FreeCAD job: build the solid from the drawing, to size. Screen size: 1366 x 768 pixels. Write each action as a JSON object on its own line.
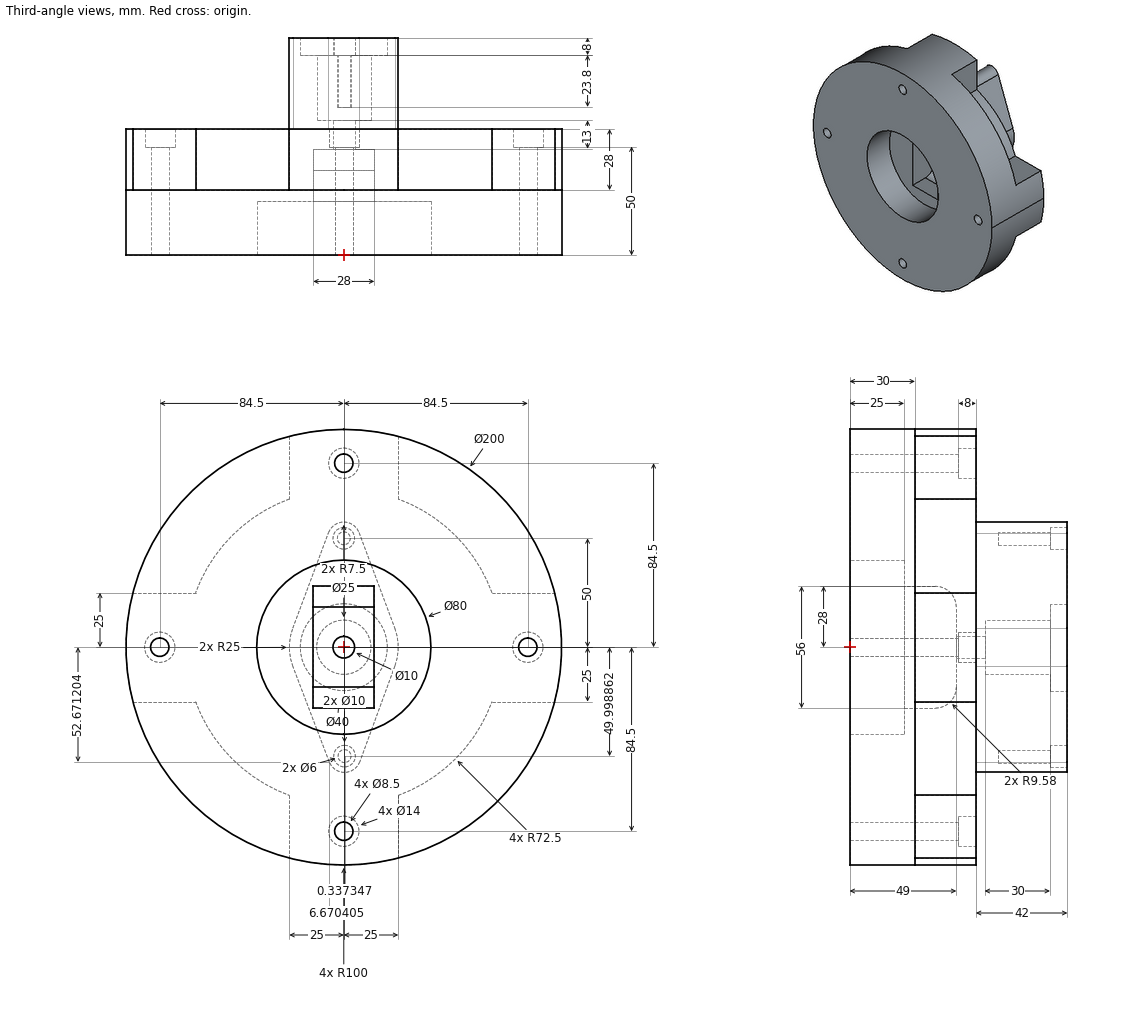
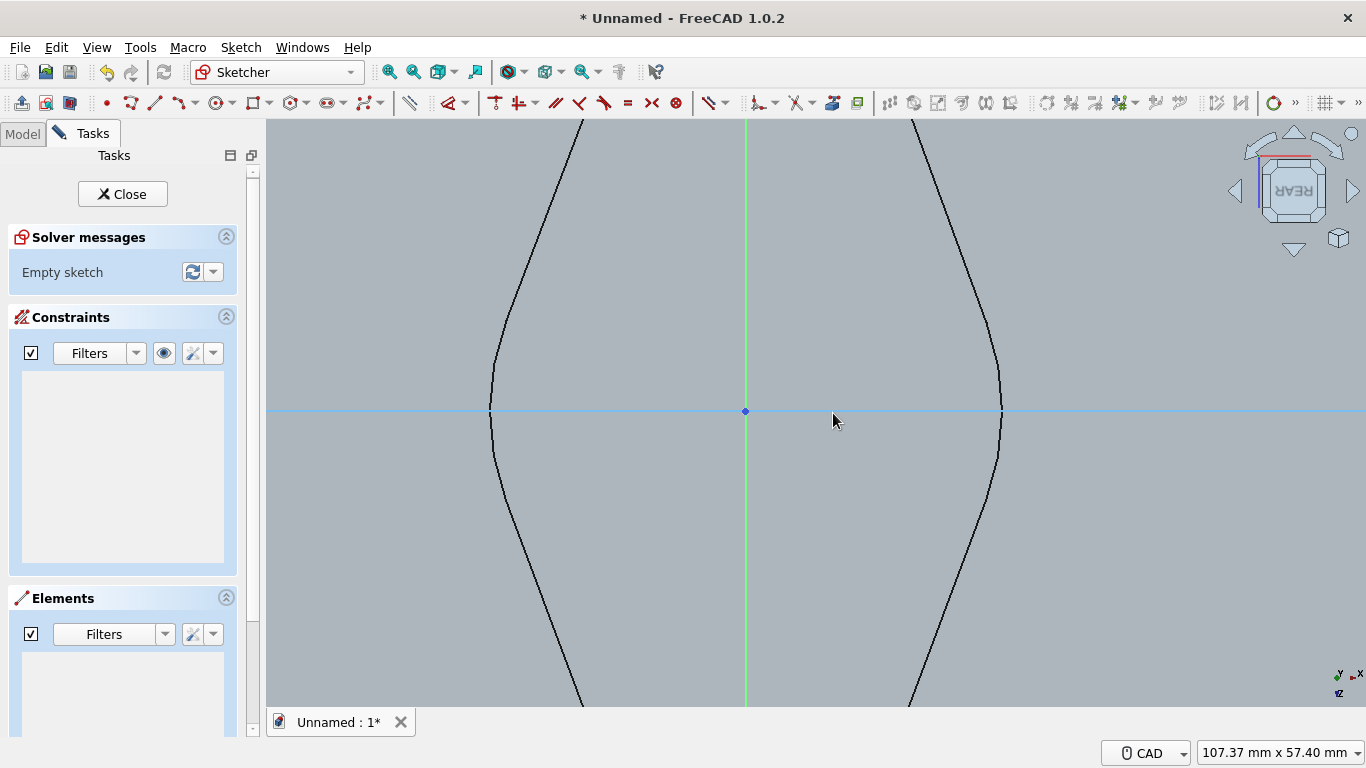
{"action": "key", "text": "g c"}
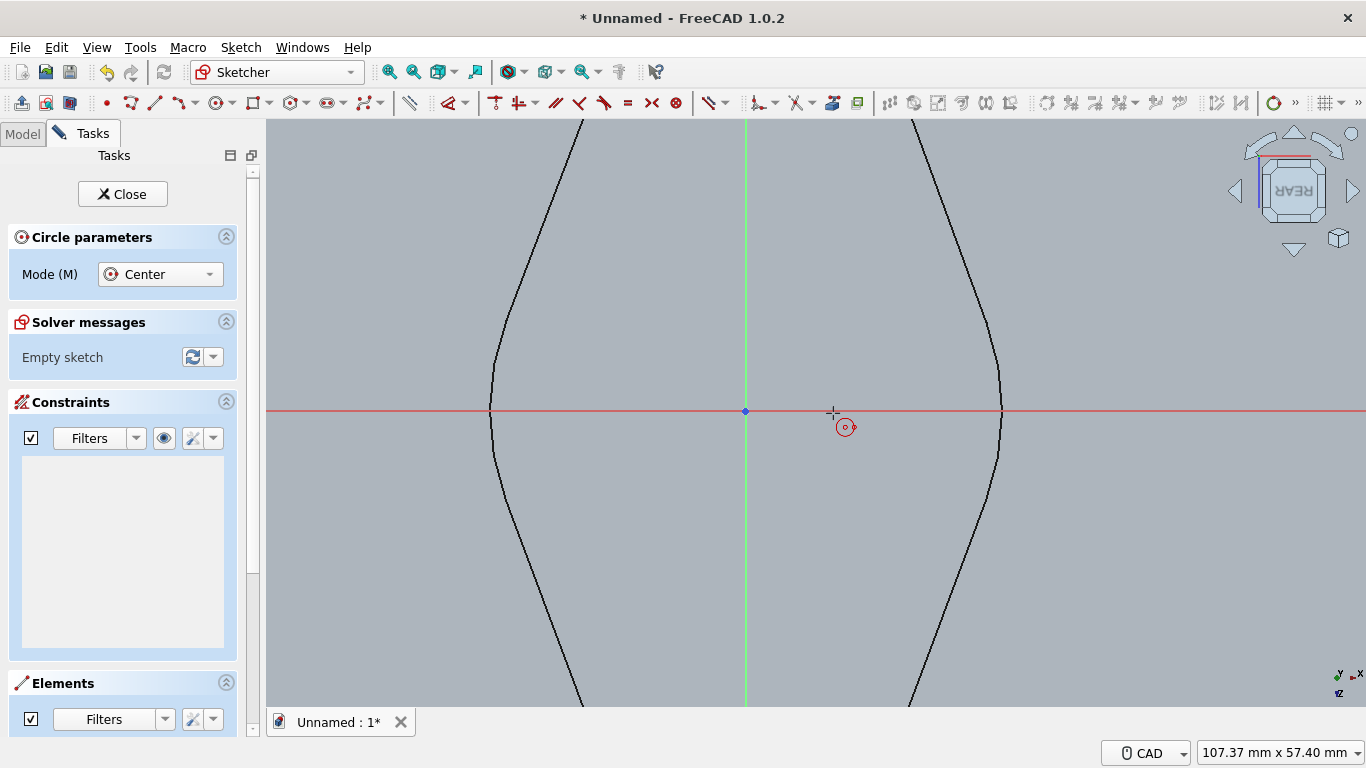
{"action": "left_click", "coordinate": [746, 411]}
{"action": "left_click", "coordinate": [891, 266]}
{"action": "key", "text": "Escape"}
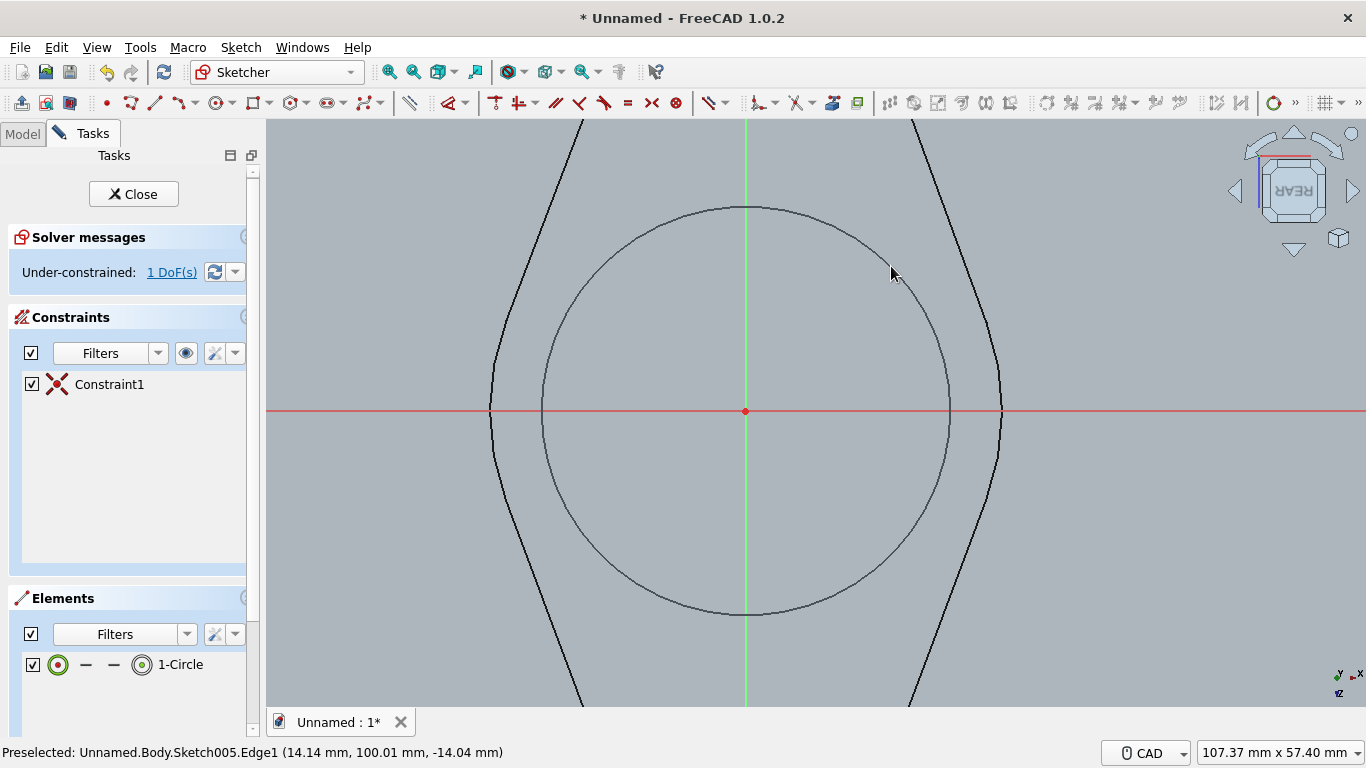
{"action": "key", "text": "d"}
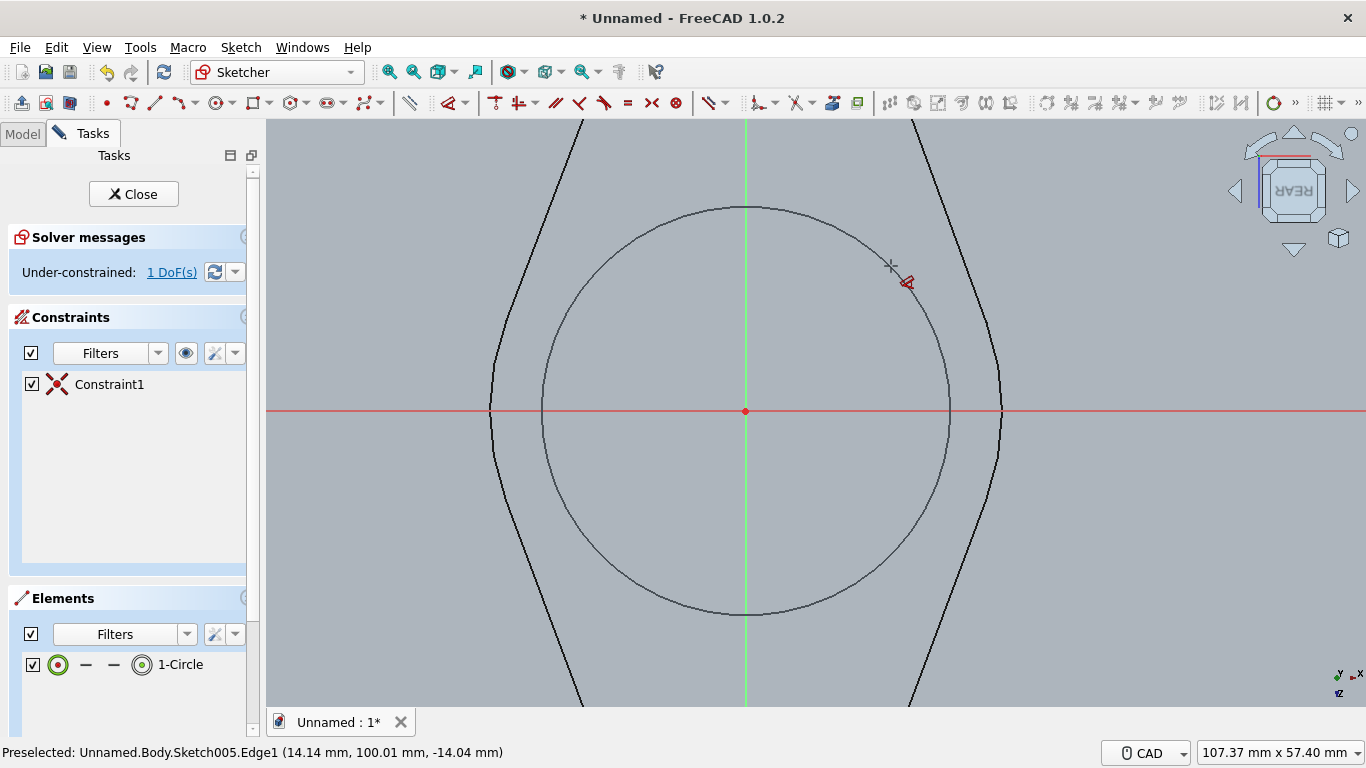
{"action": "left_click", "coordinate": [890, 266]}
{"action": "left_click", "coordinate": [913, 243]}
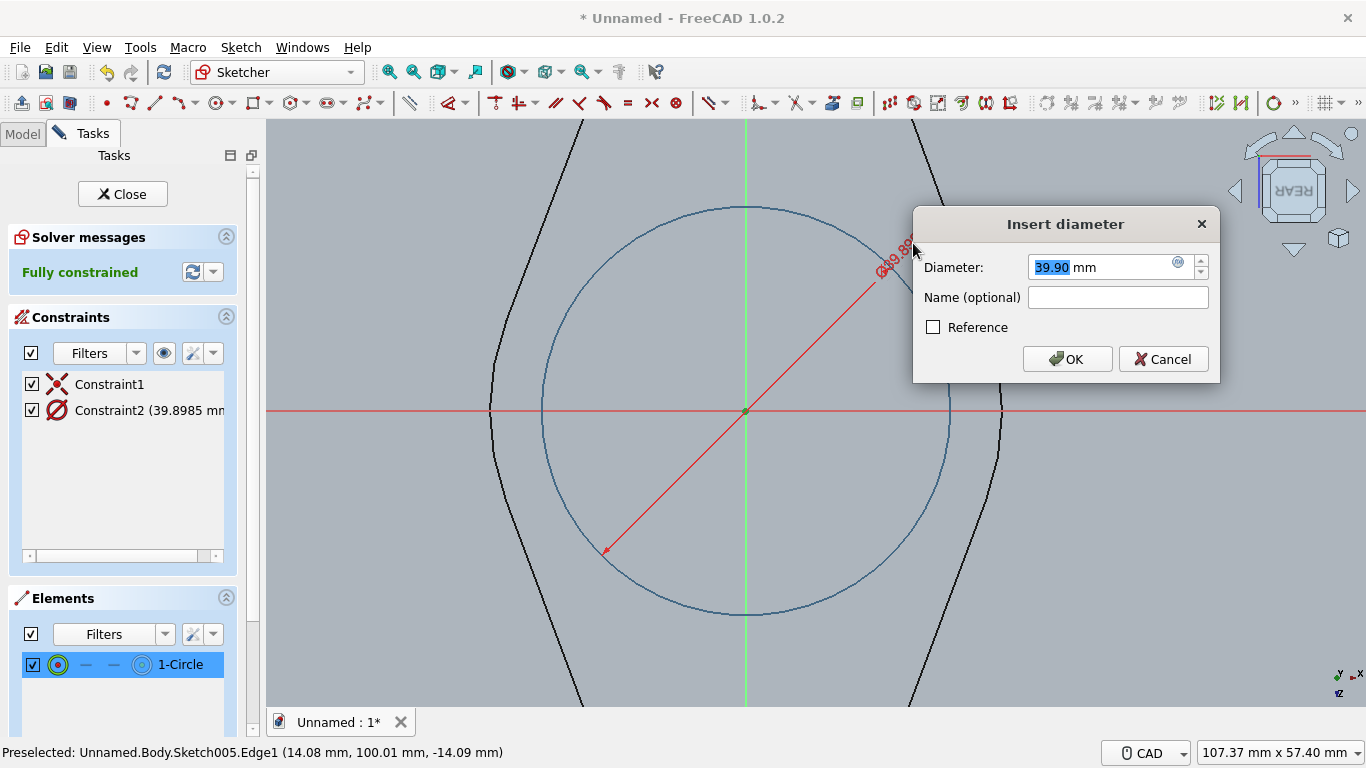
{"action": "type", "text": "40"}
{"action": "key", "text": "Return"}
{"action": "key", "text": "Escape"}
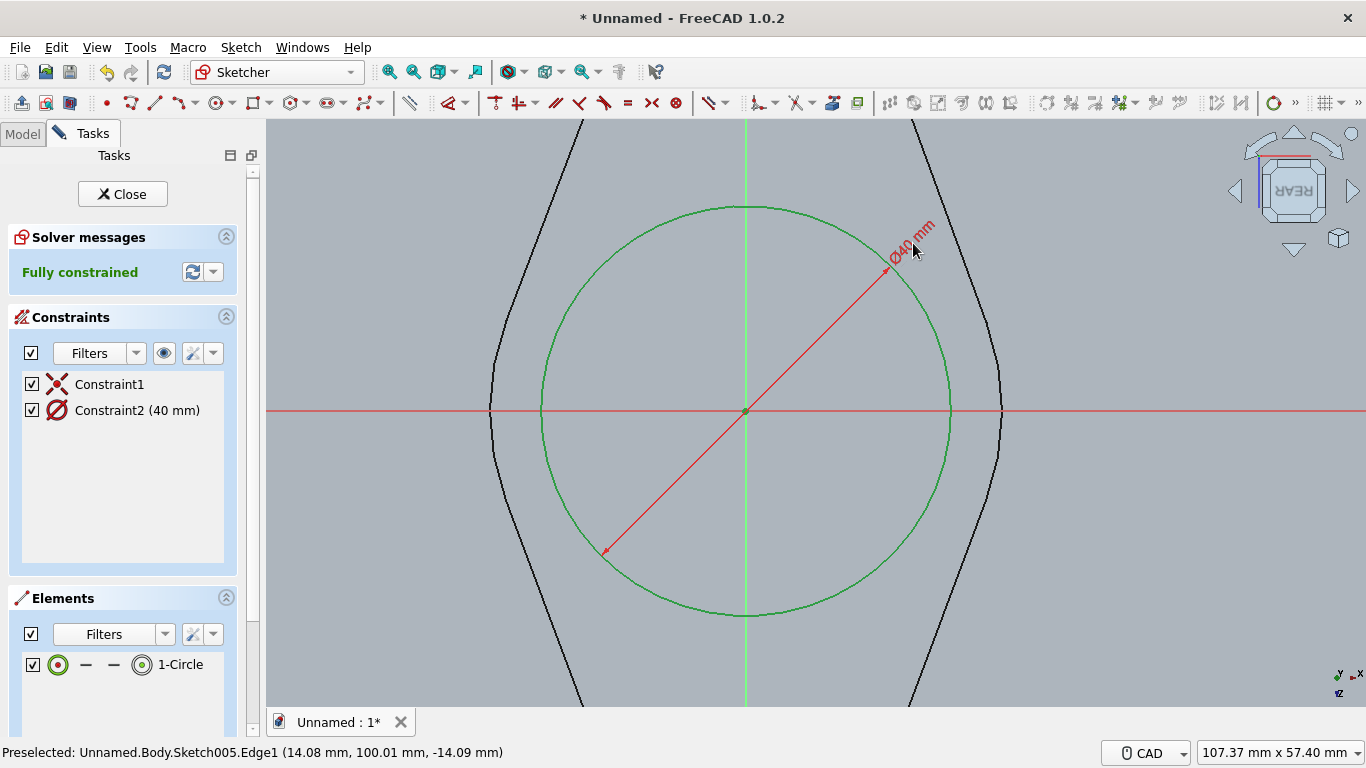
{"action": "left_click", "coordinate": [123, 194]}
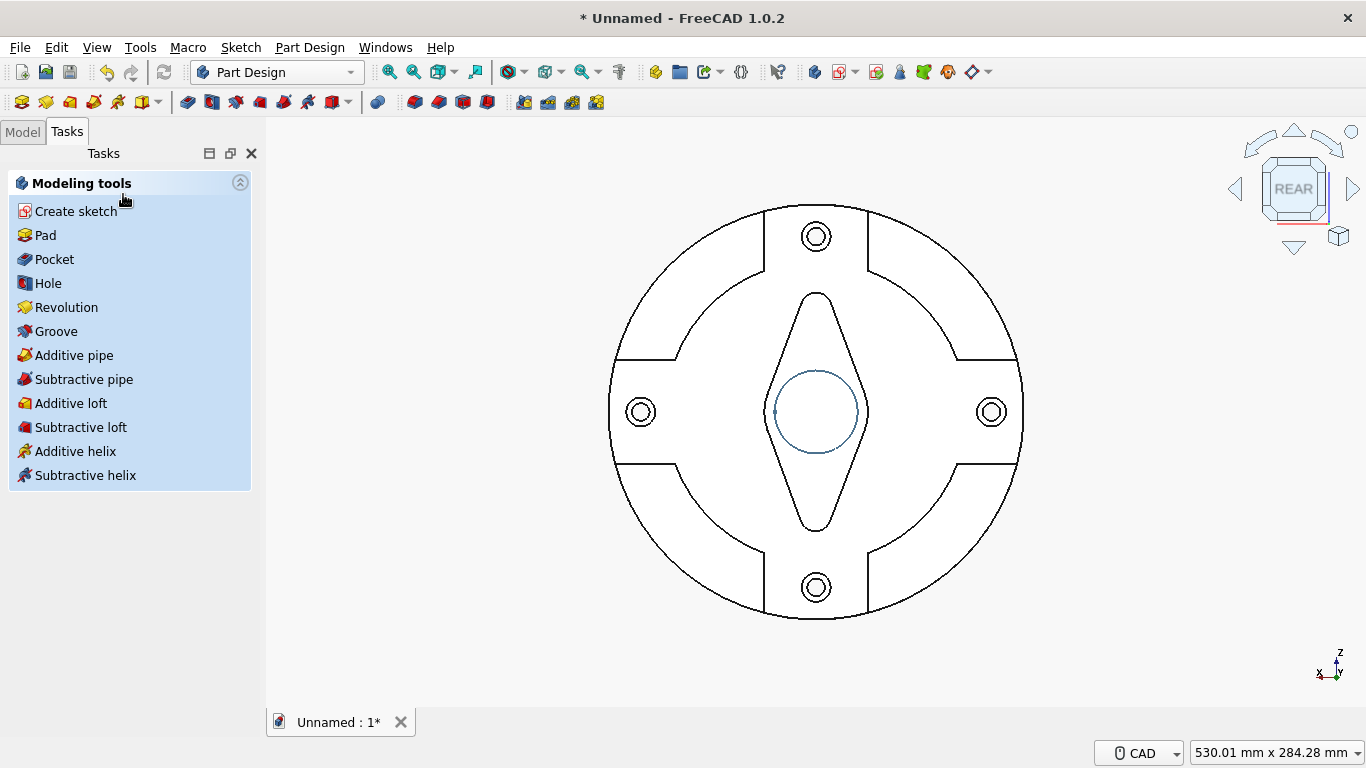
{"action": "left_click", "coordinate": [188, 102]}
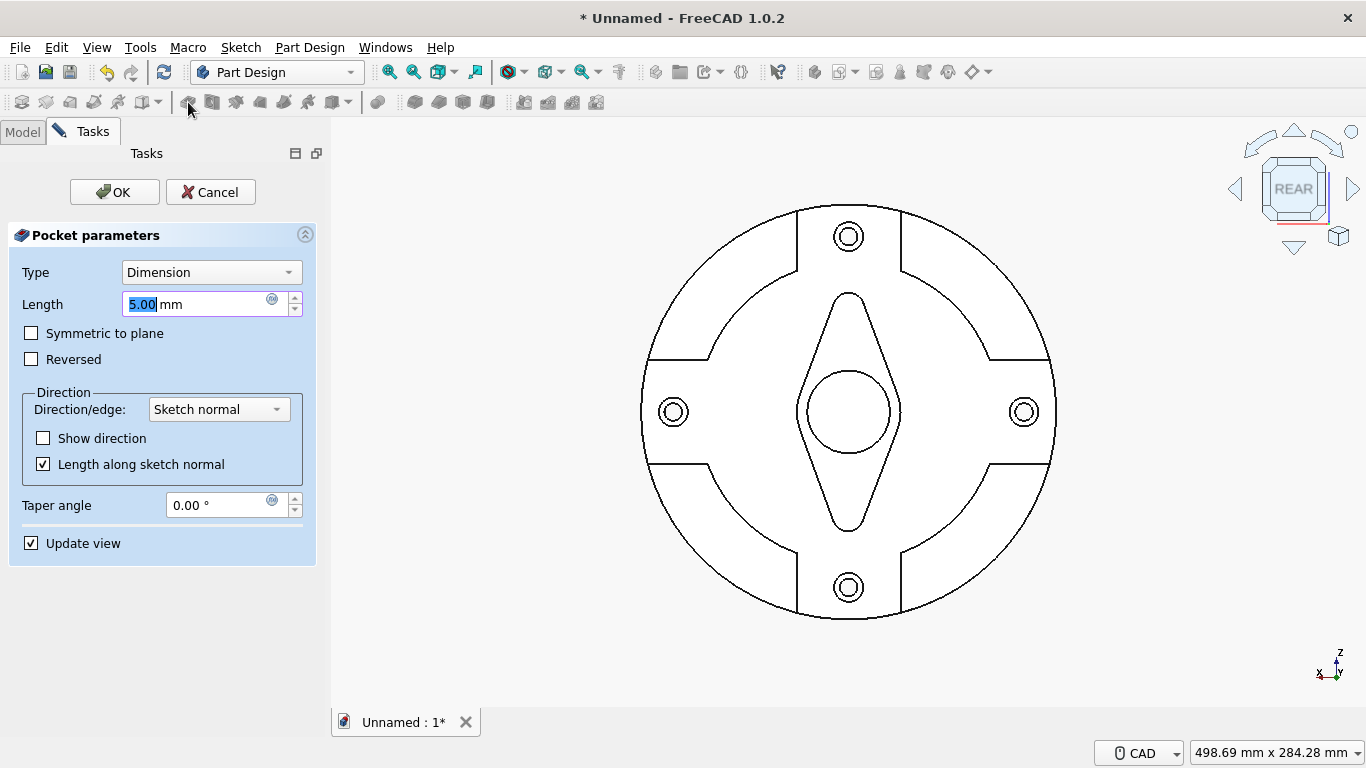
{"action": "type", "text": "8"}
{"action": "key", "text": "Tab"}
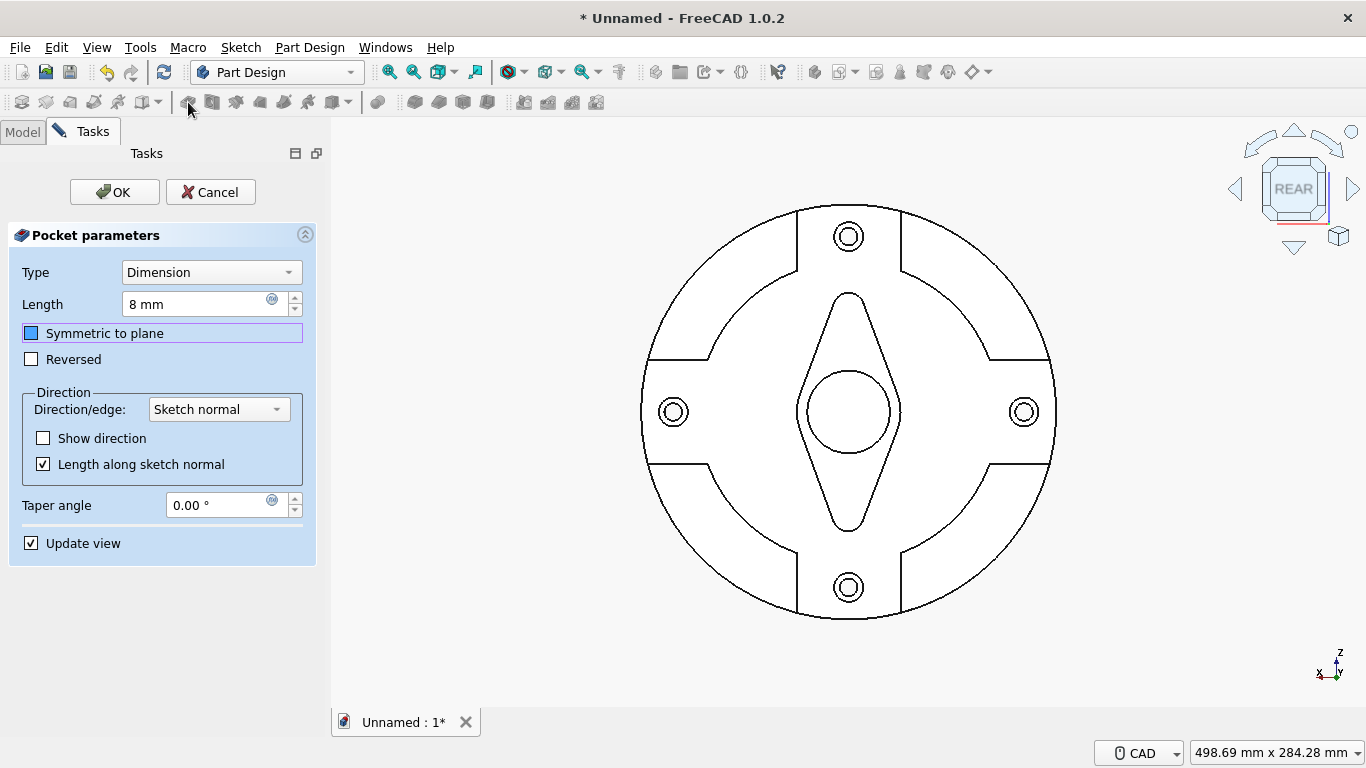
{"action": "left_click", "coordinate": [115, 192]}